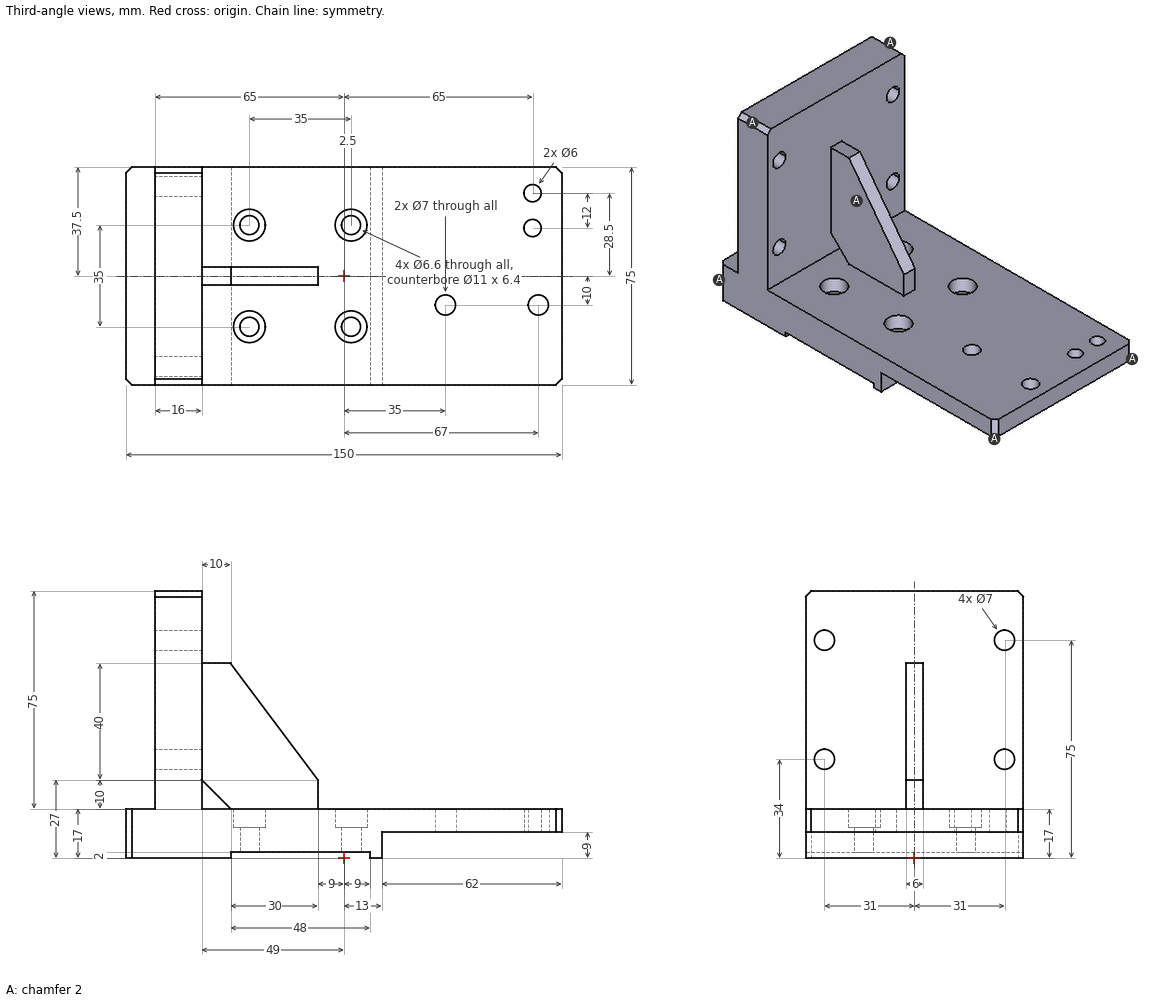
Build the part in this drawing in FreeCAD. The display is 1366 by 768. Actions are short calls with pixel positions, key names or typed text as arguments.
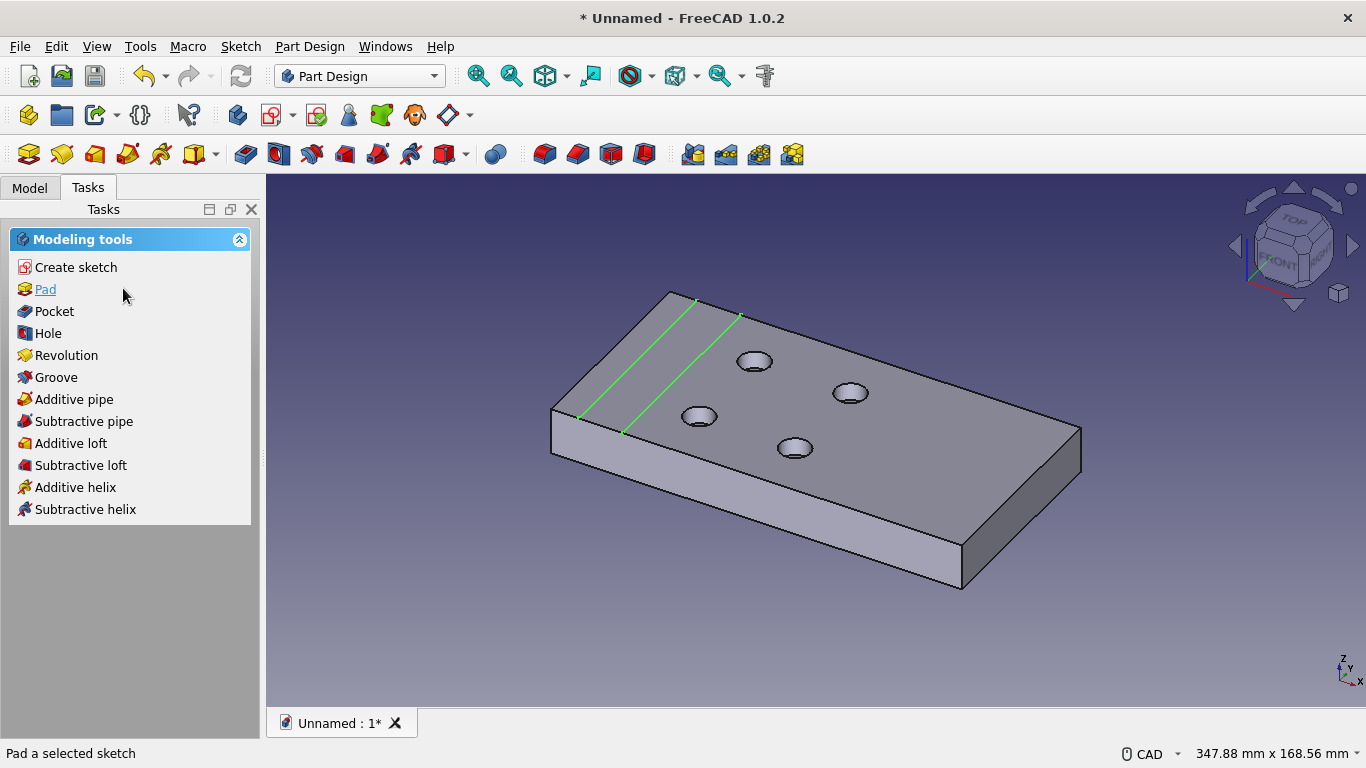
click(29, 154)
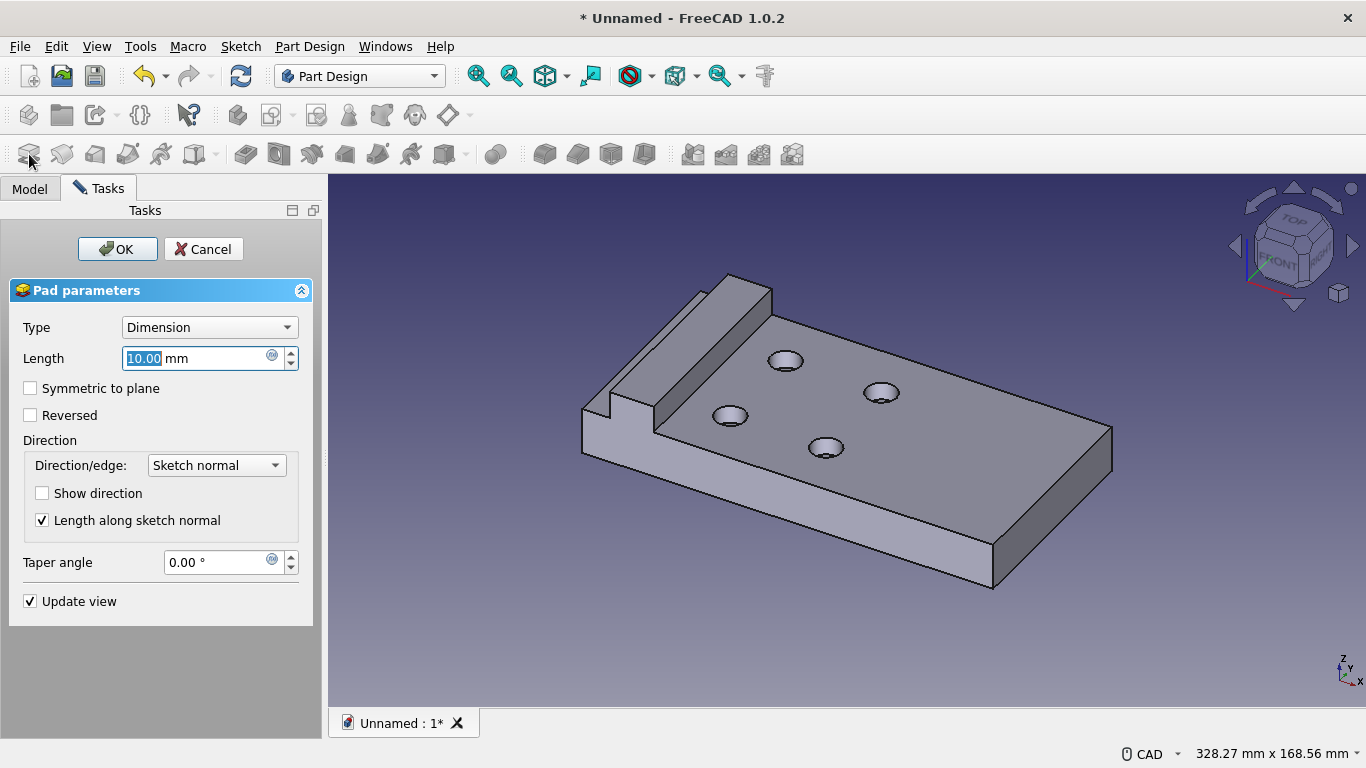
text(75)
key(Tab)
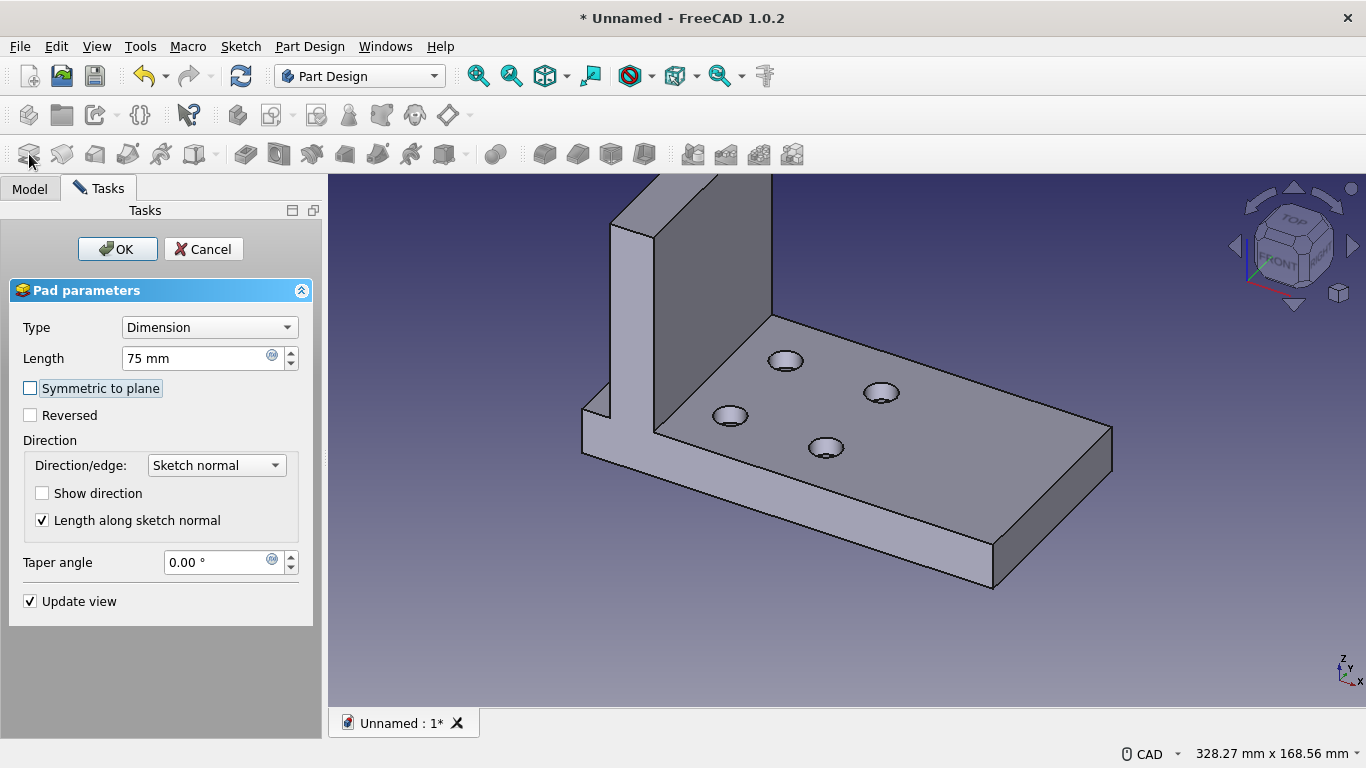
click(118, 249)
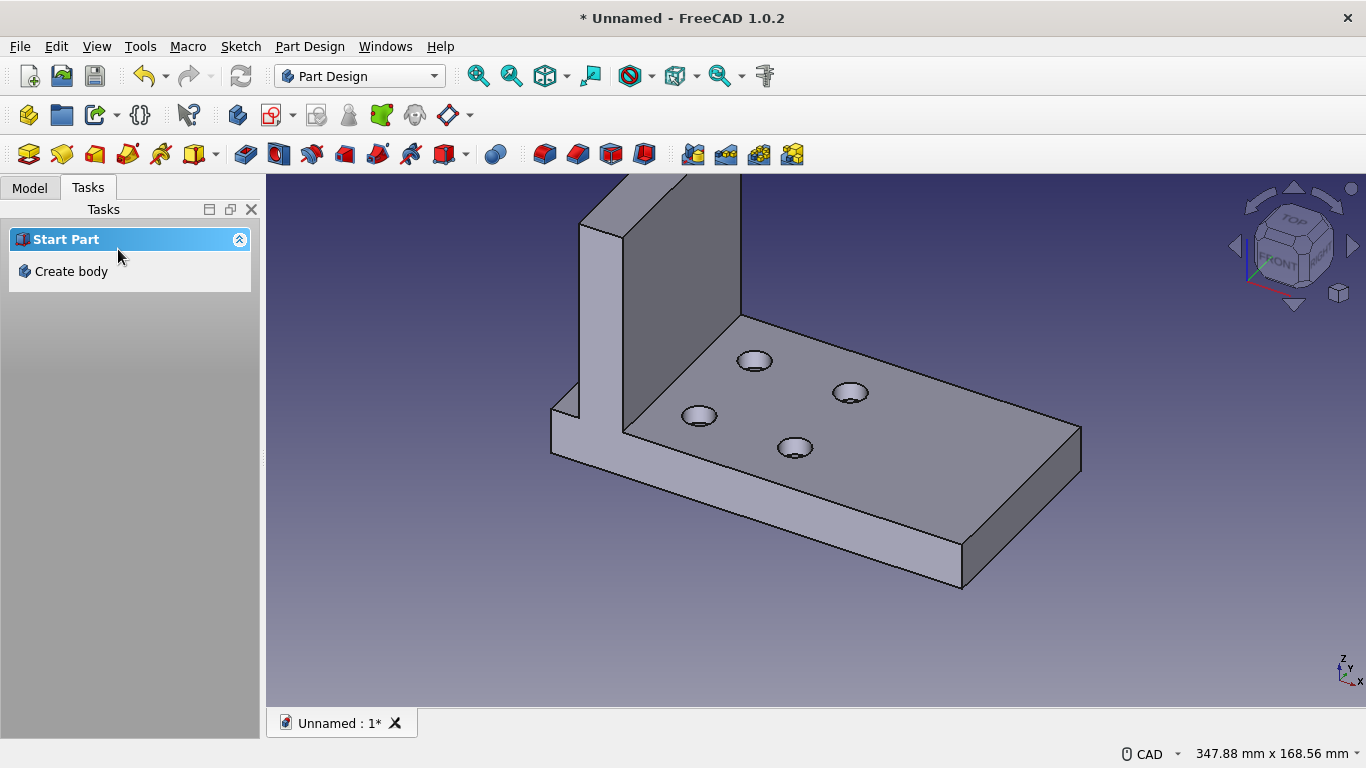
click(479, 76)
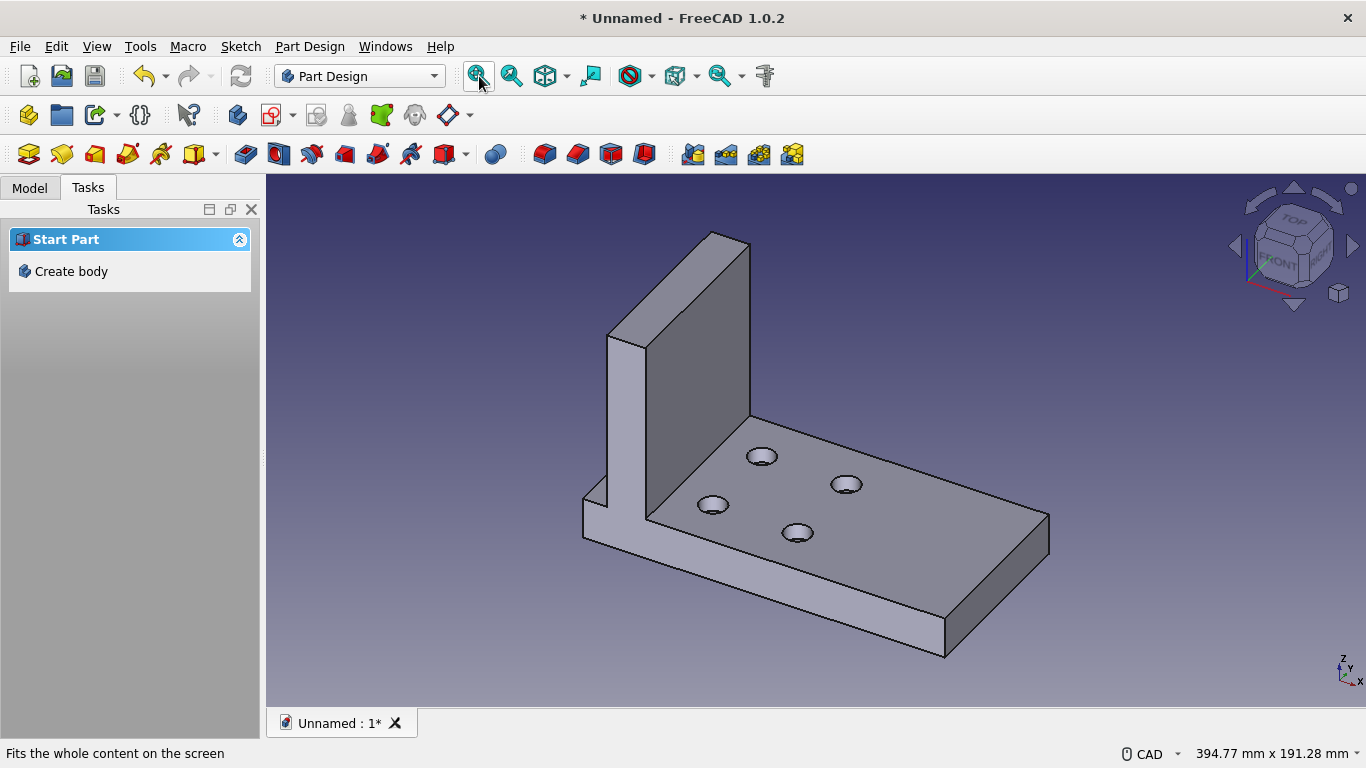
click(698, 381)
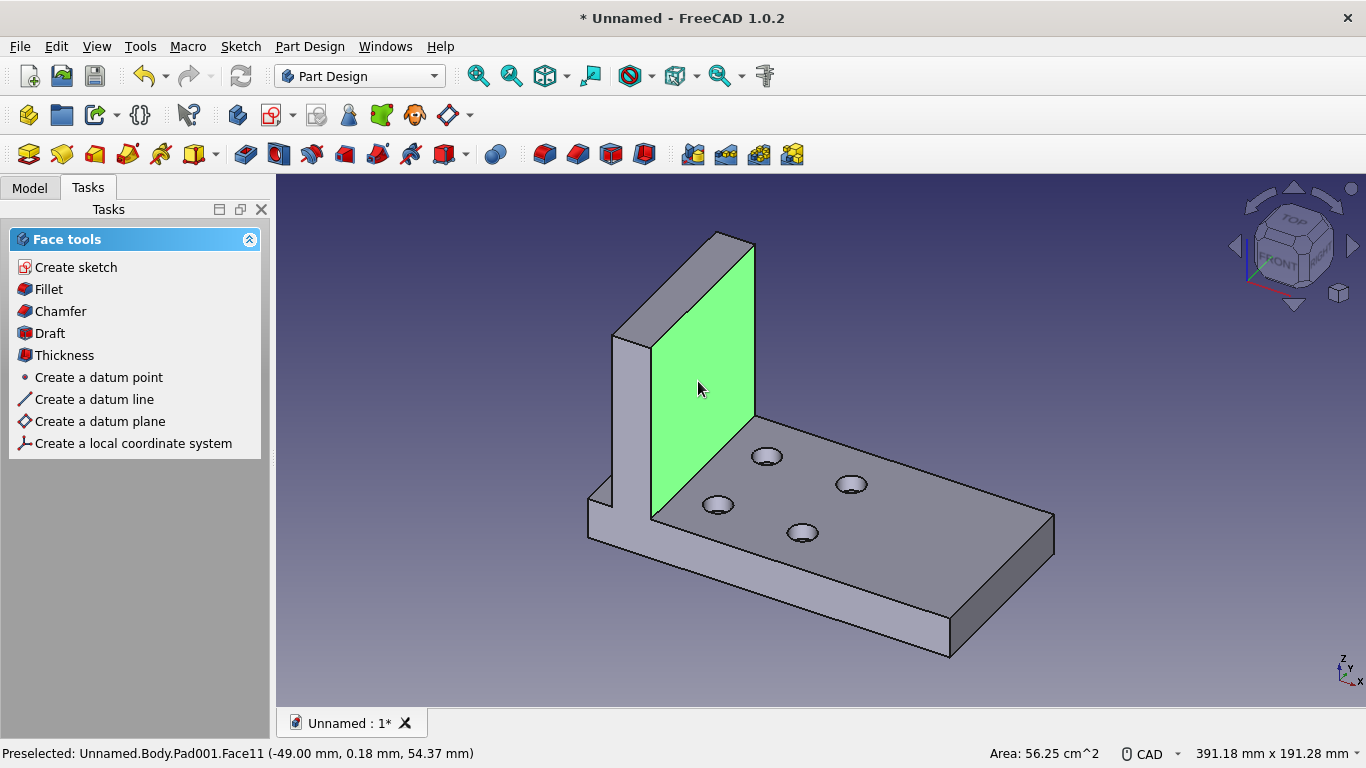
click(270, 116)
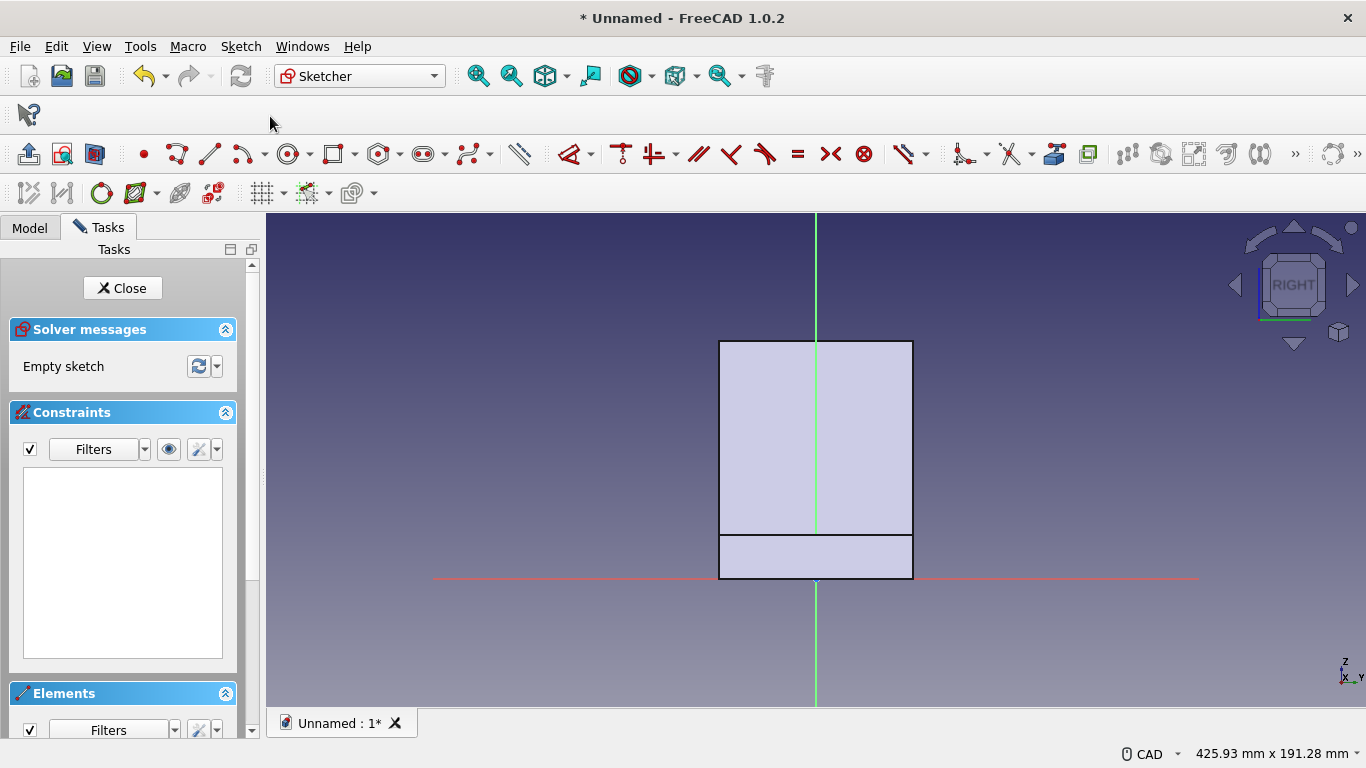
click(95, 154)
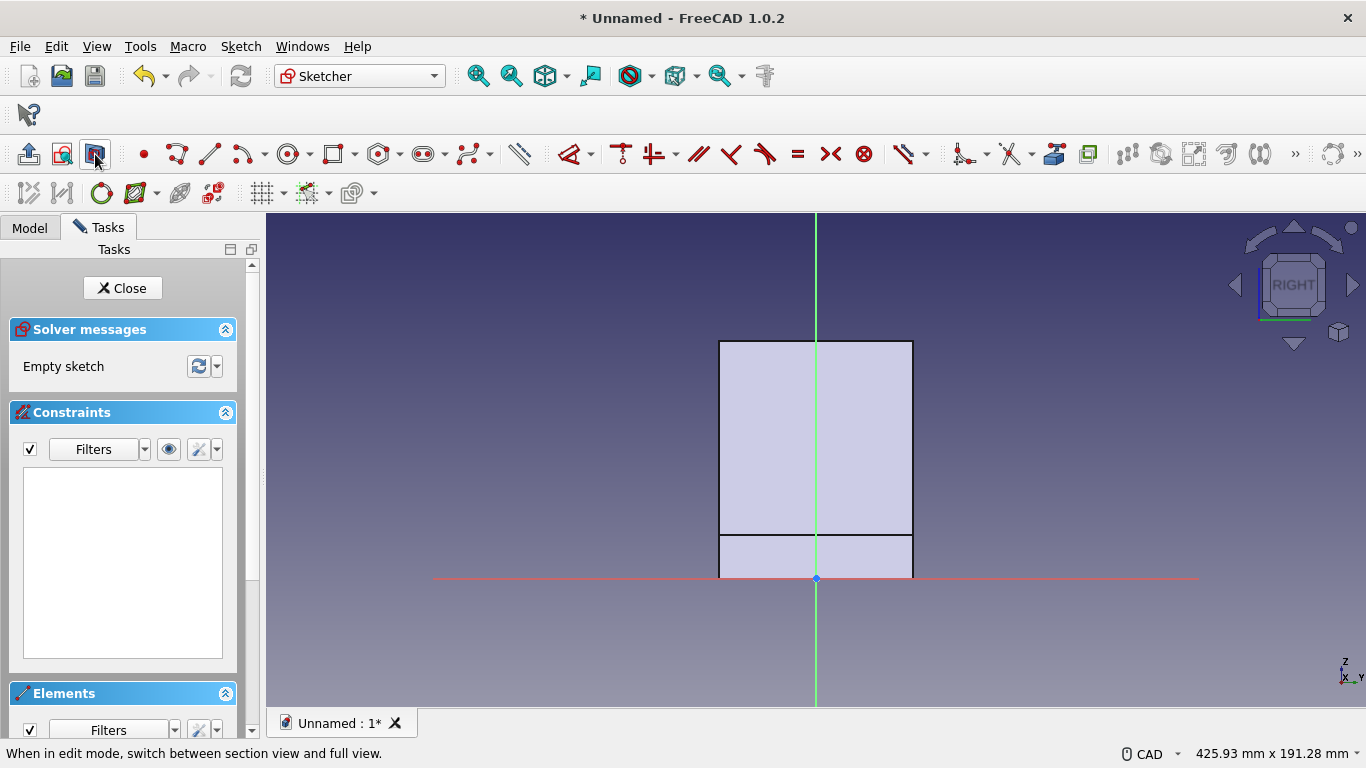
scroll(955, 513, up, 2)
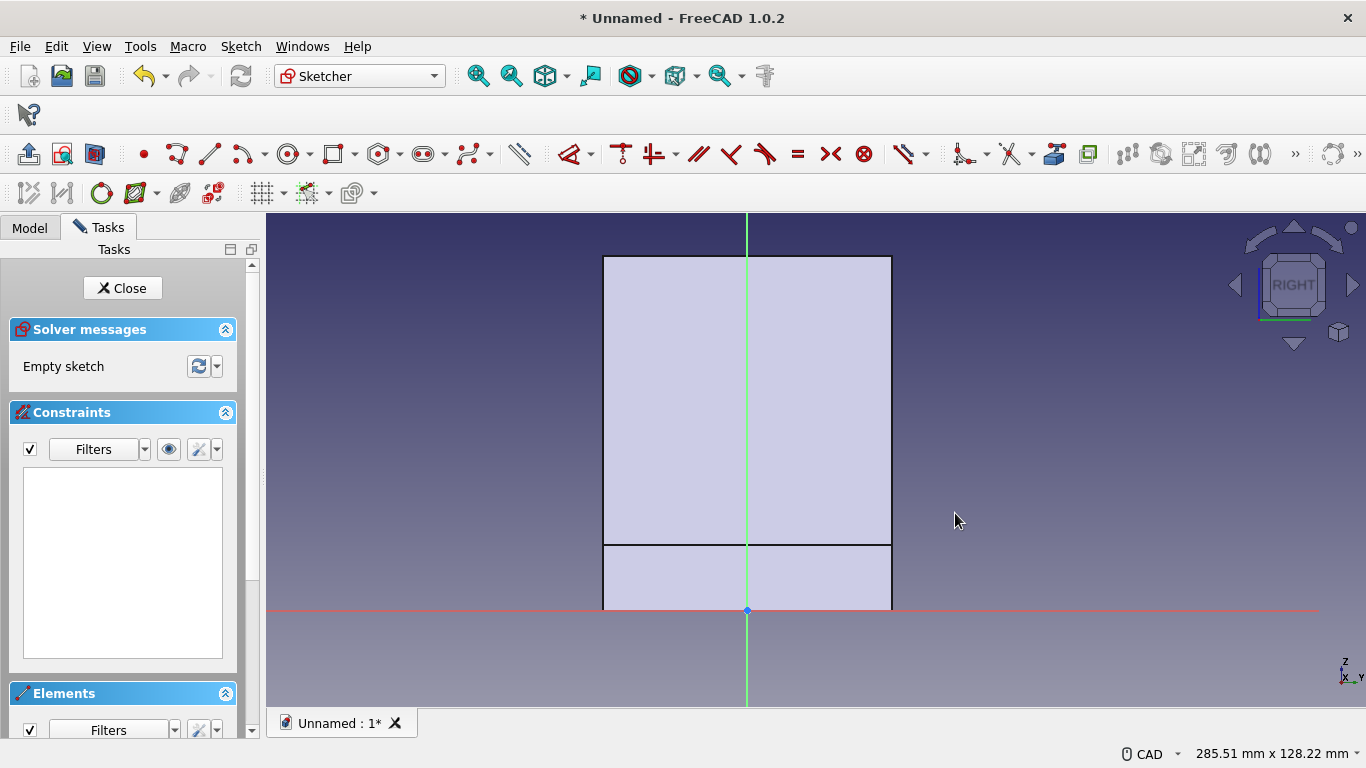
click(288, 154)